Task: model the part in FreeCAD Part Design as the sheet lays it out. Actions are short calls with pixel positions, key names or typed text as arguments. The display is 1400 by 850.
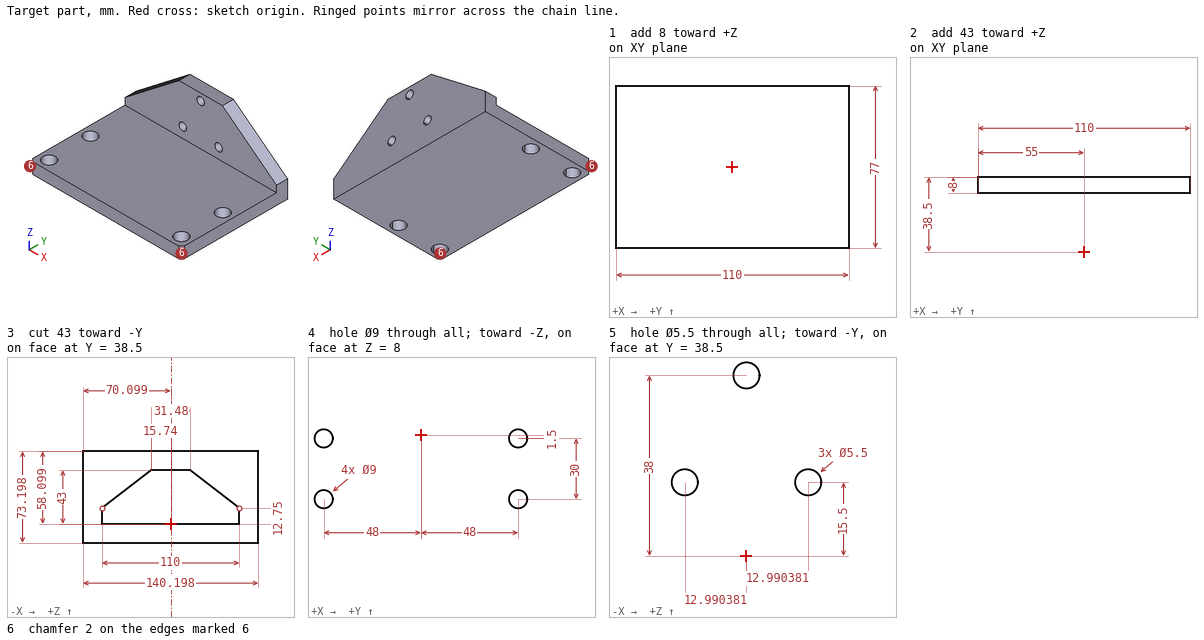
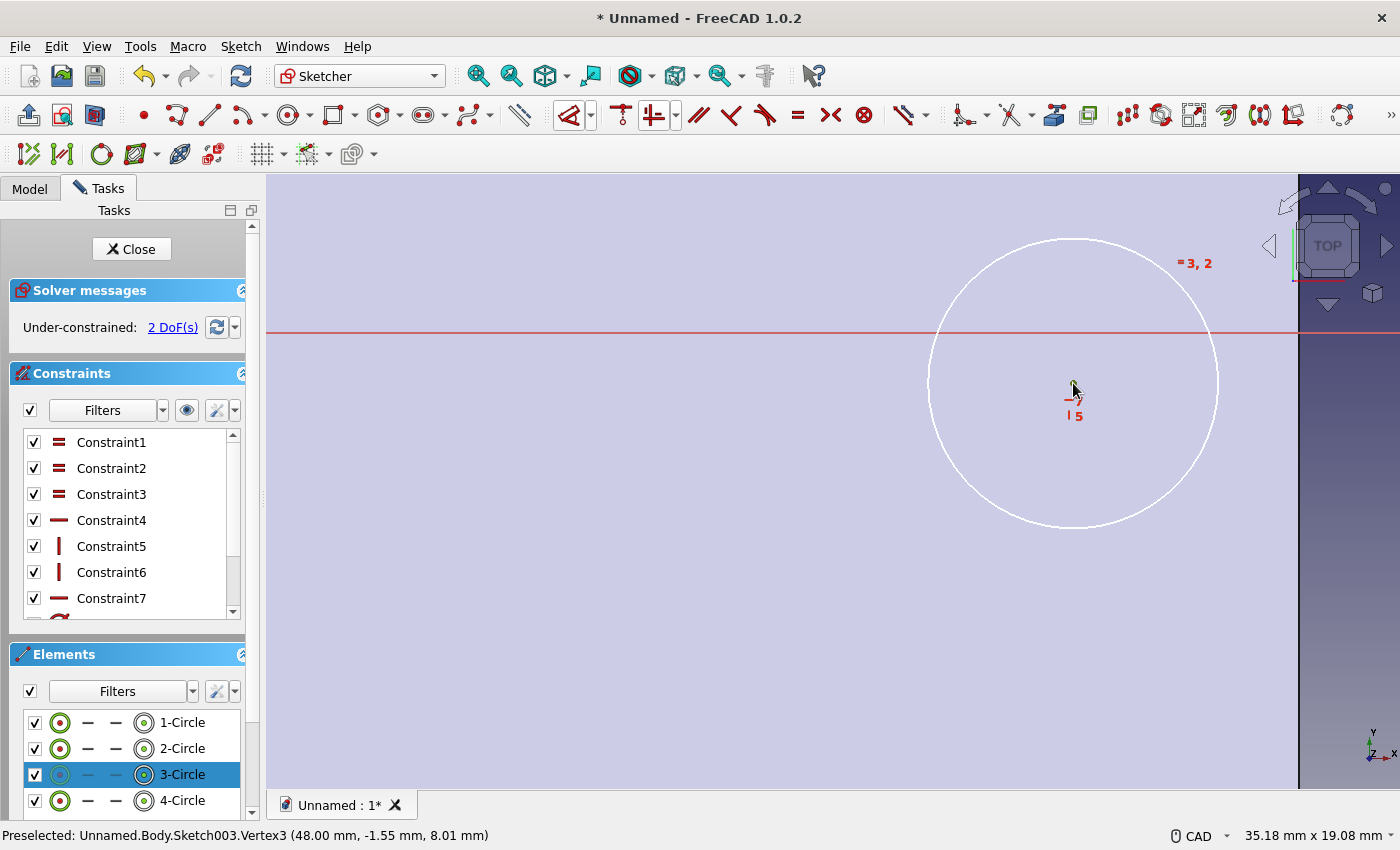
key(i)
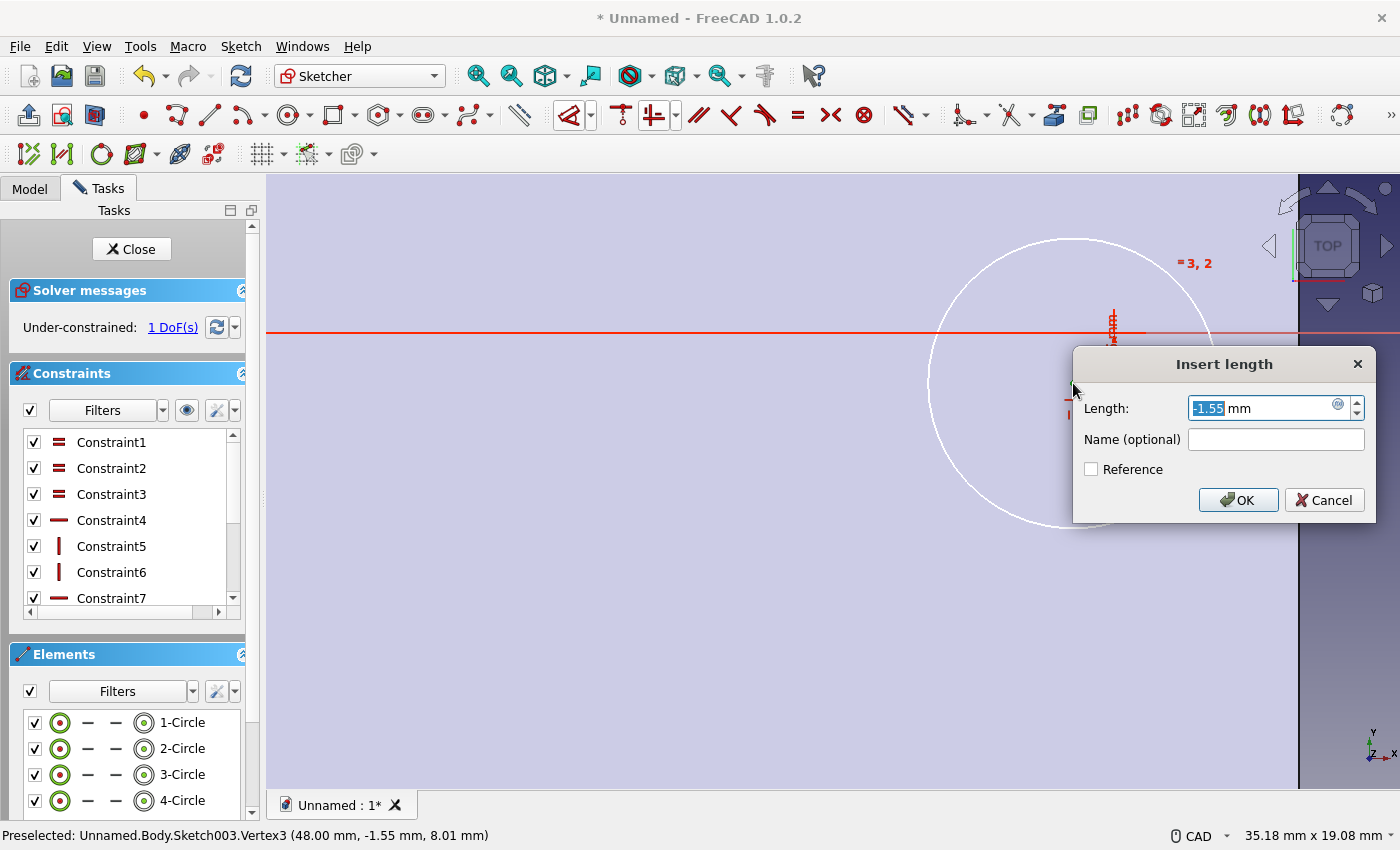
text(-1.5)
key(Return)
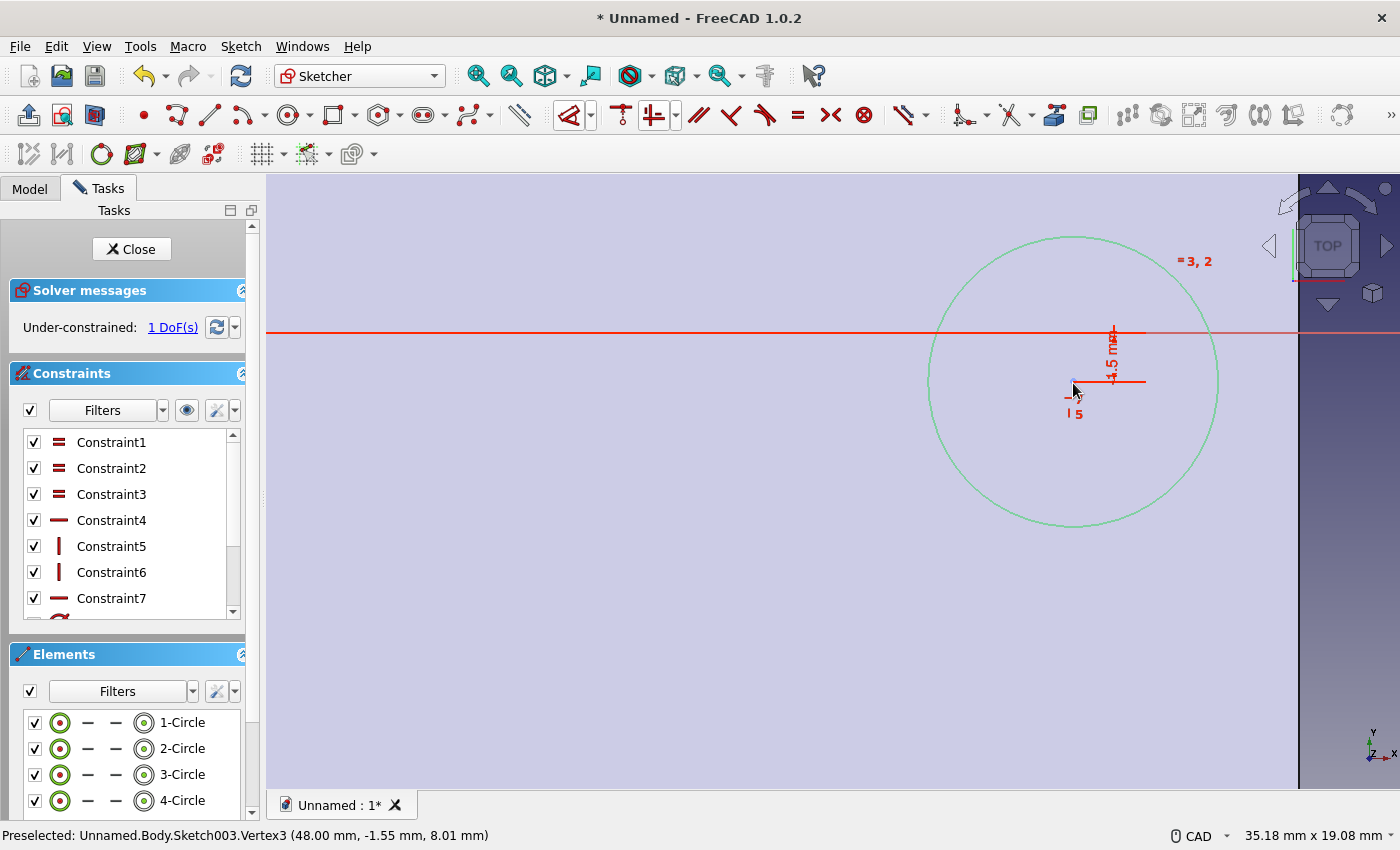
scroll(1078, 384, down, 8)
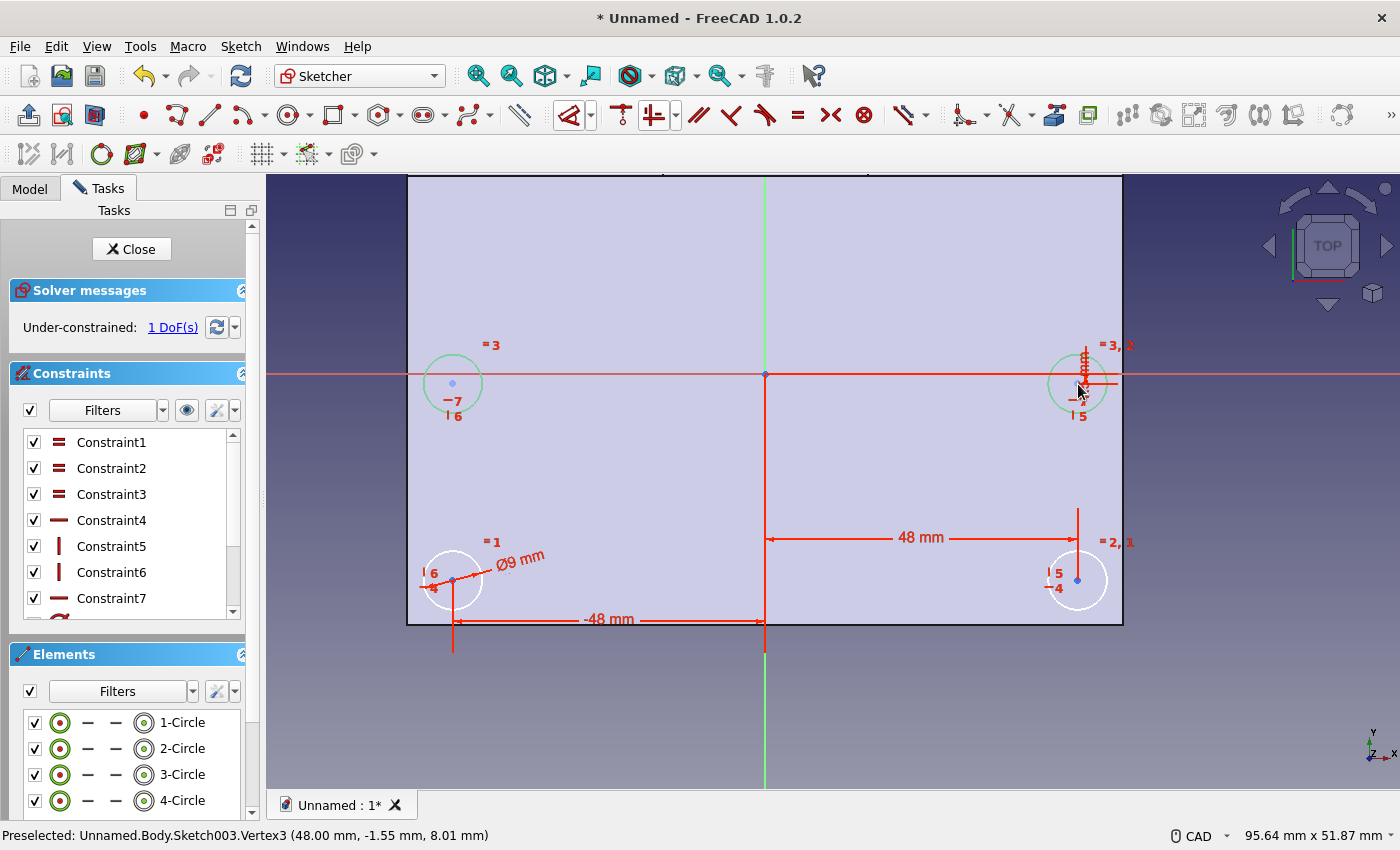
click(1078, 580)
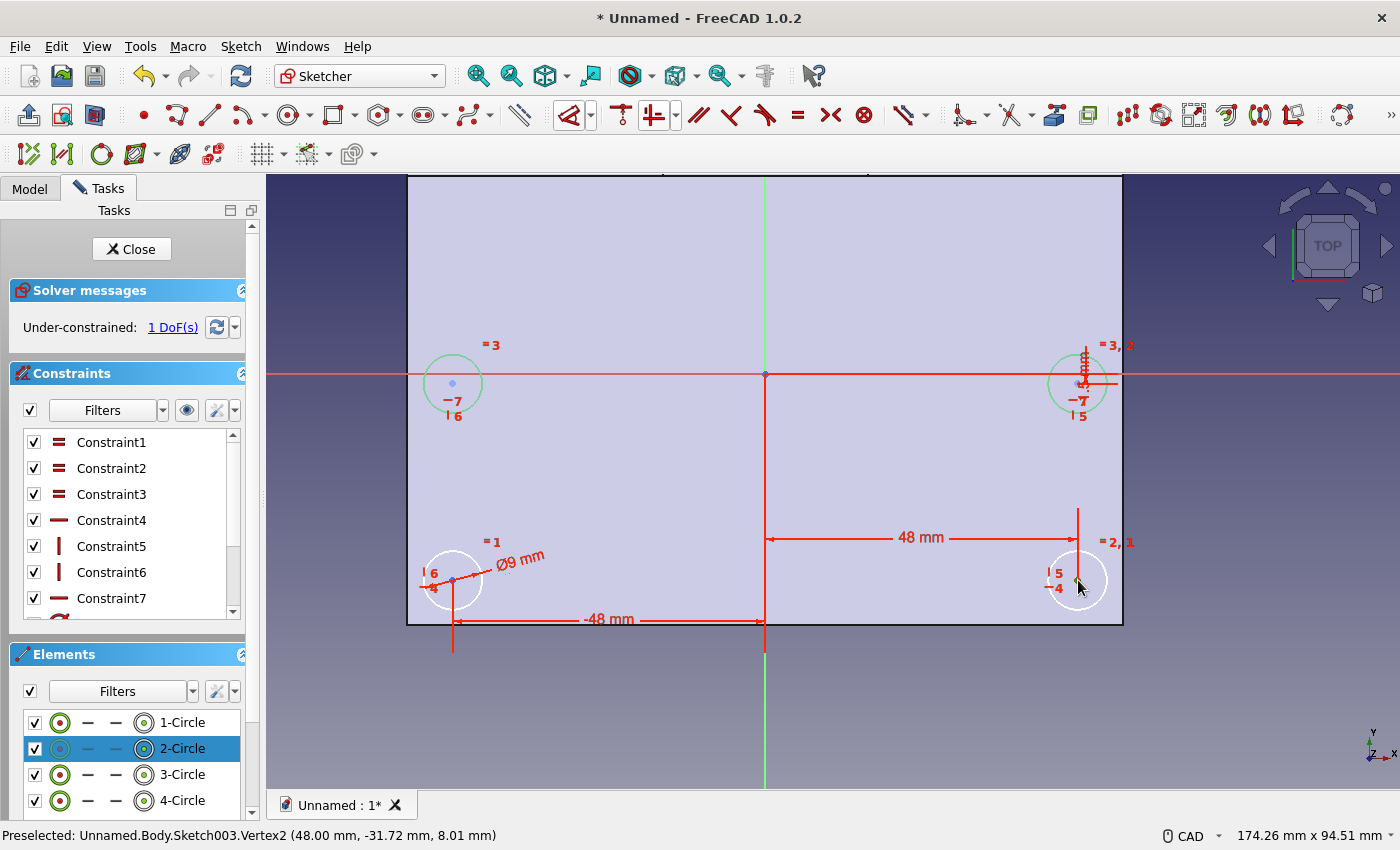
click(1078, 384)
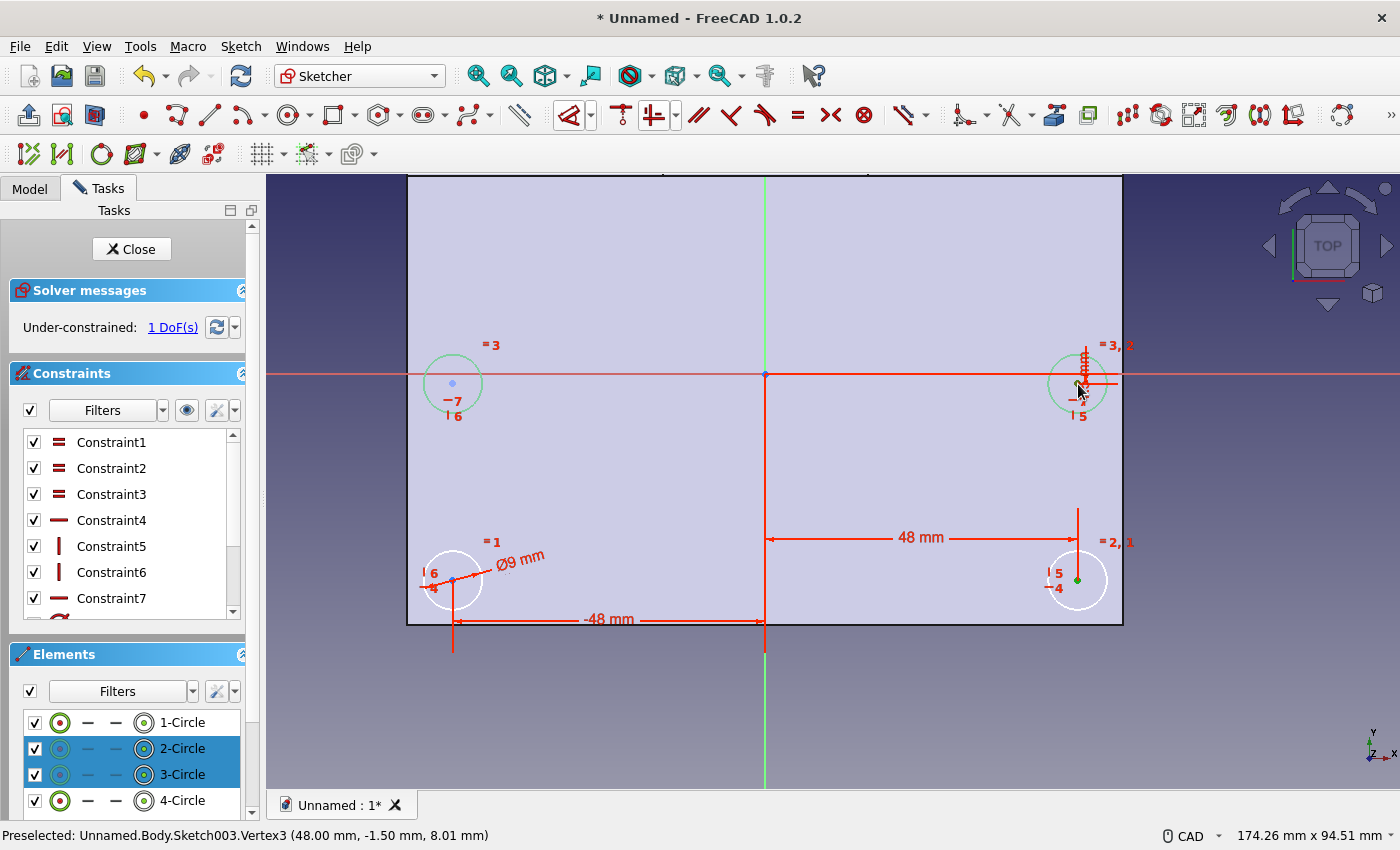
key(i)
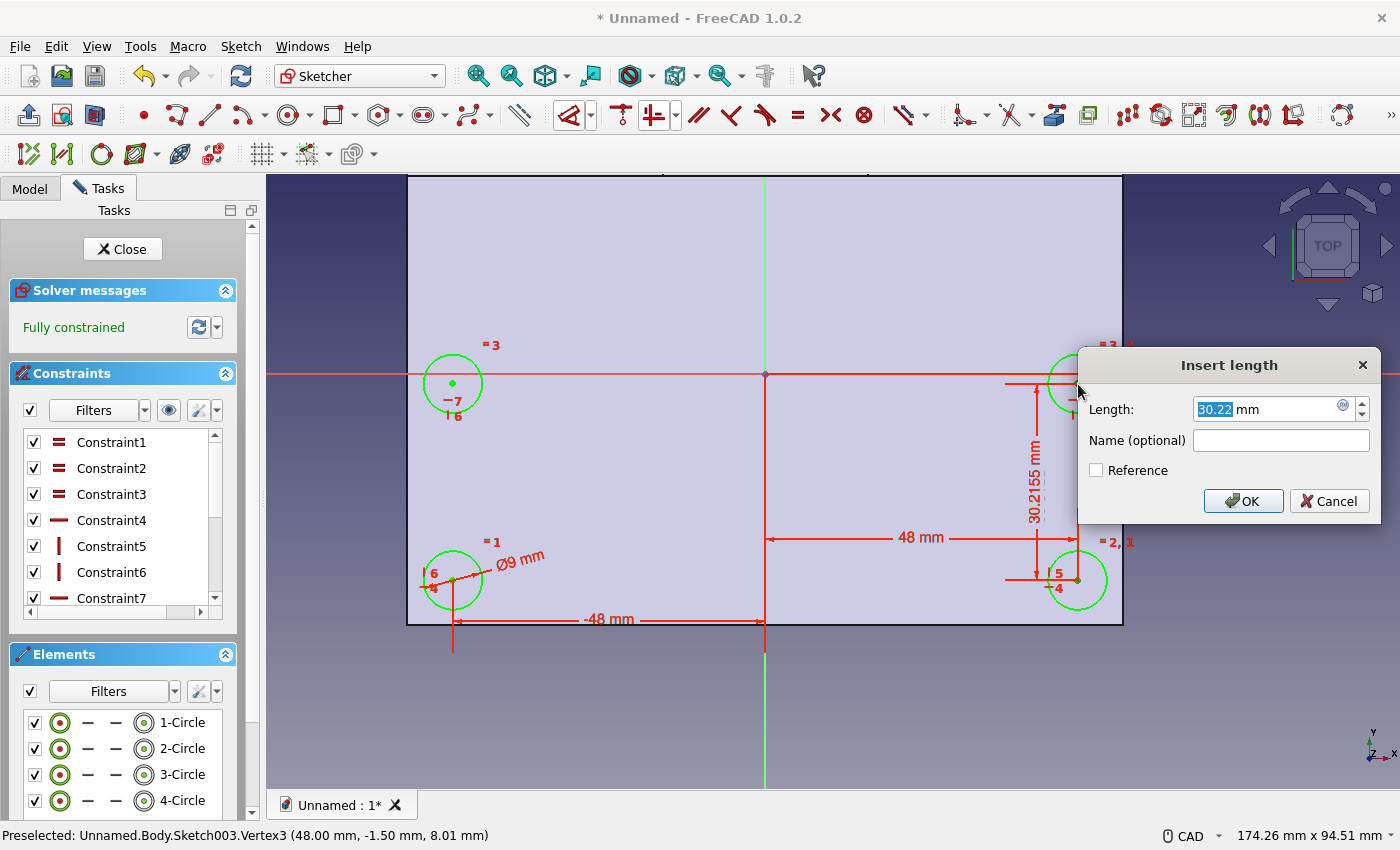
text(30)
key(Return)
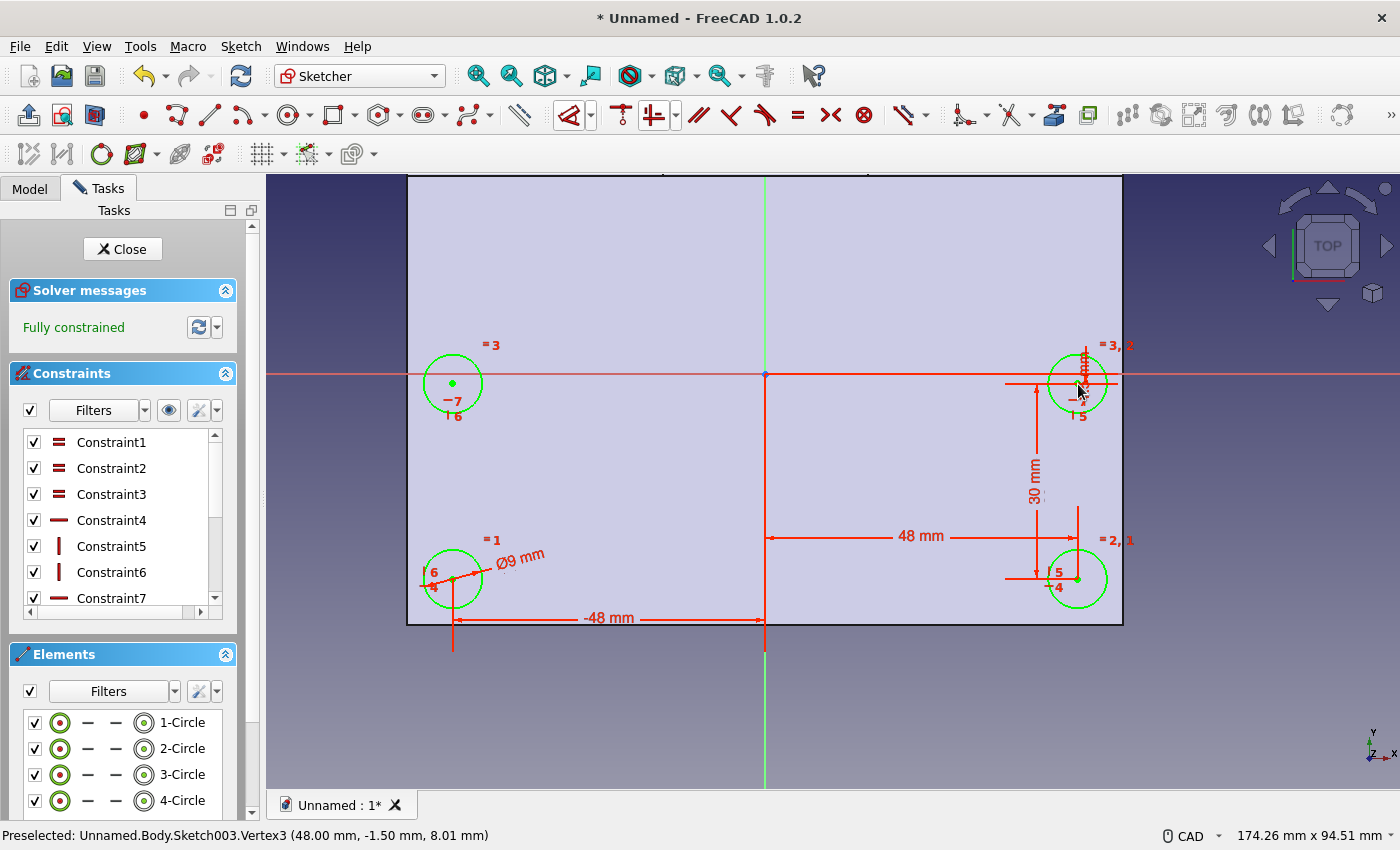
click(123, 249)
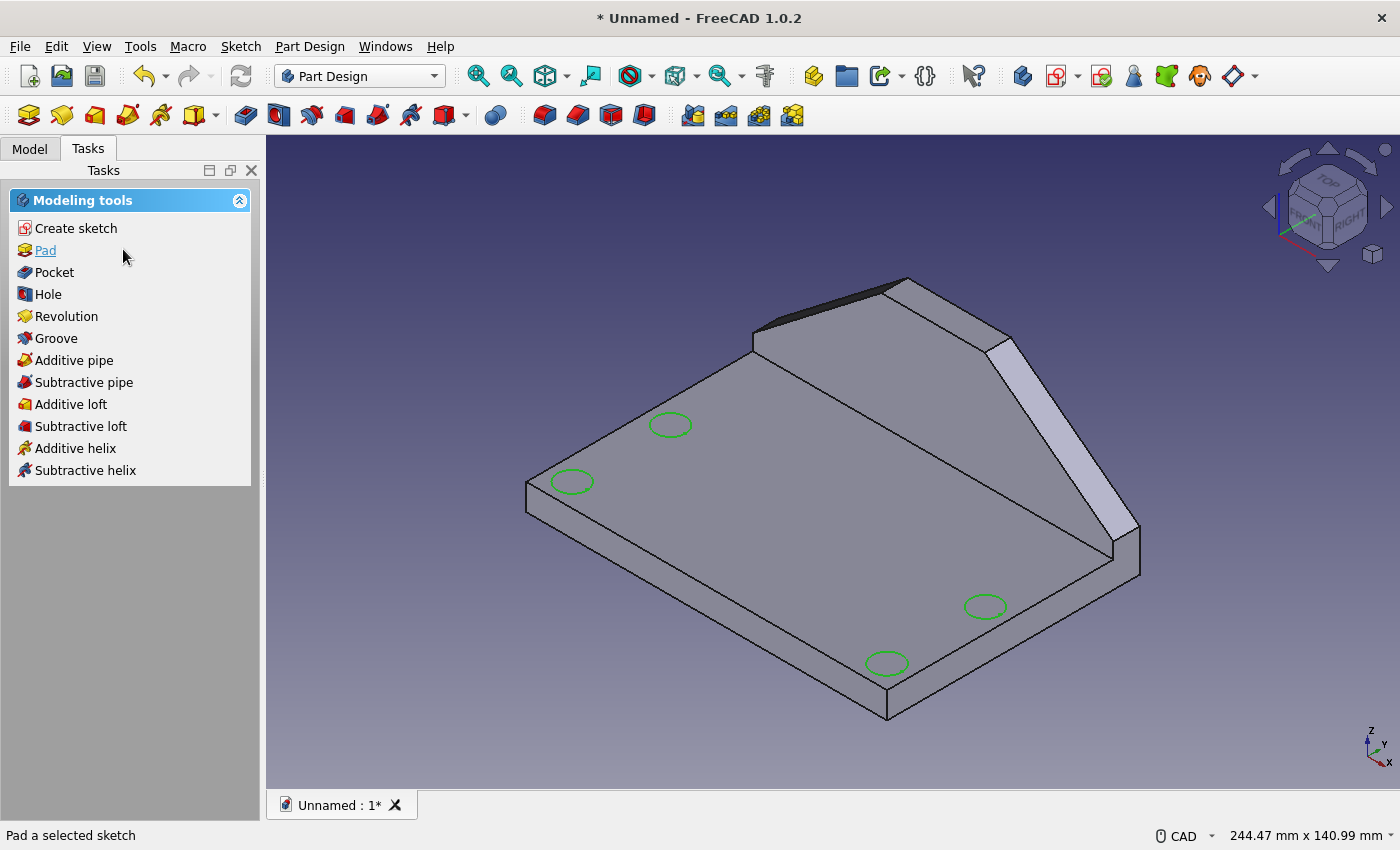
click(279, 116)